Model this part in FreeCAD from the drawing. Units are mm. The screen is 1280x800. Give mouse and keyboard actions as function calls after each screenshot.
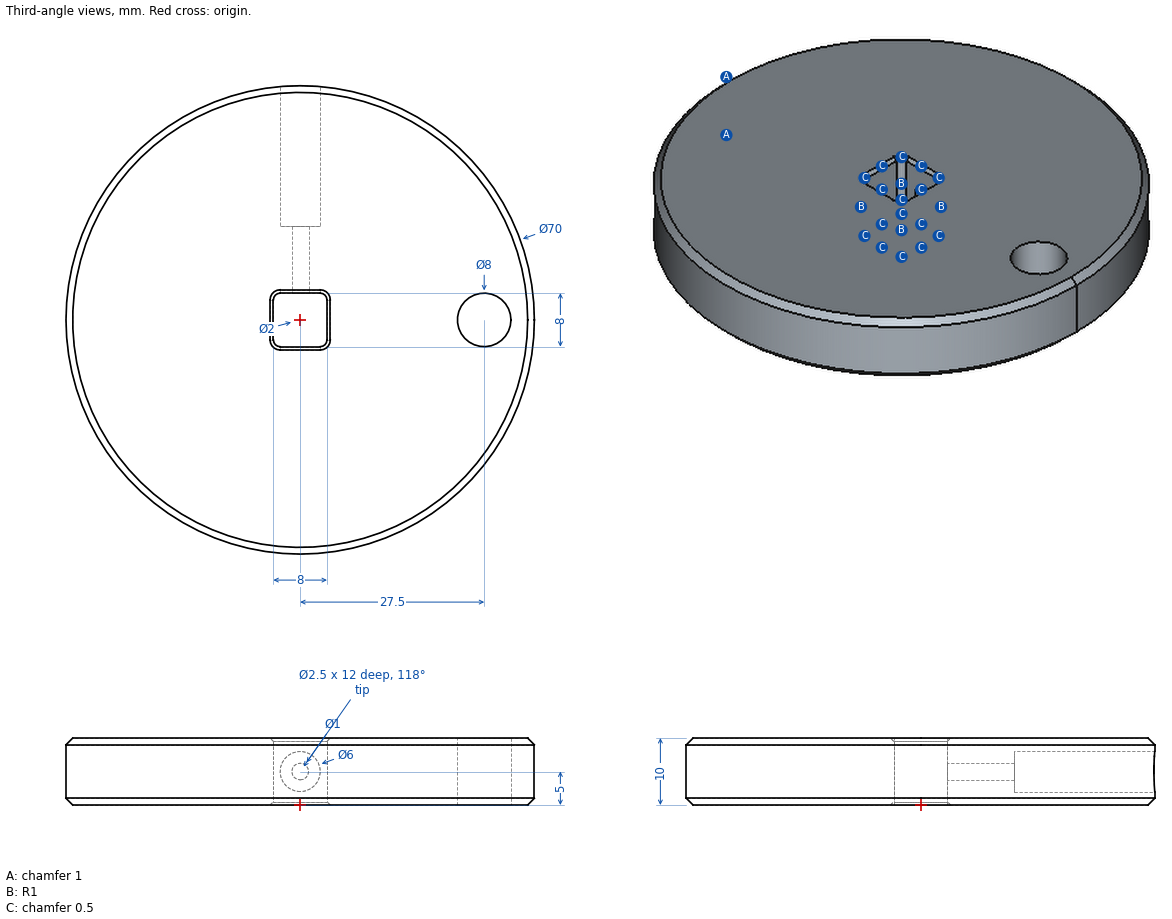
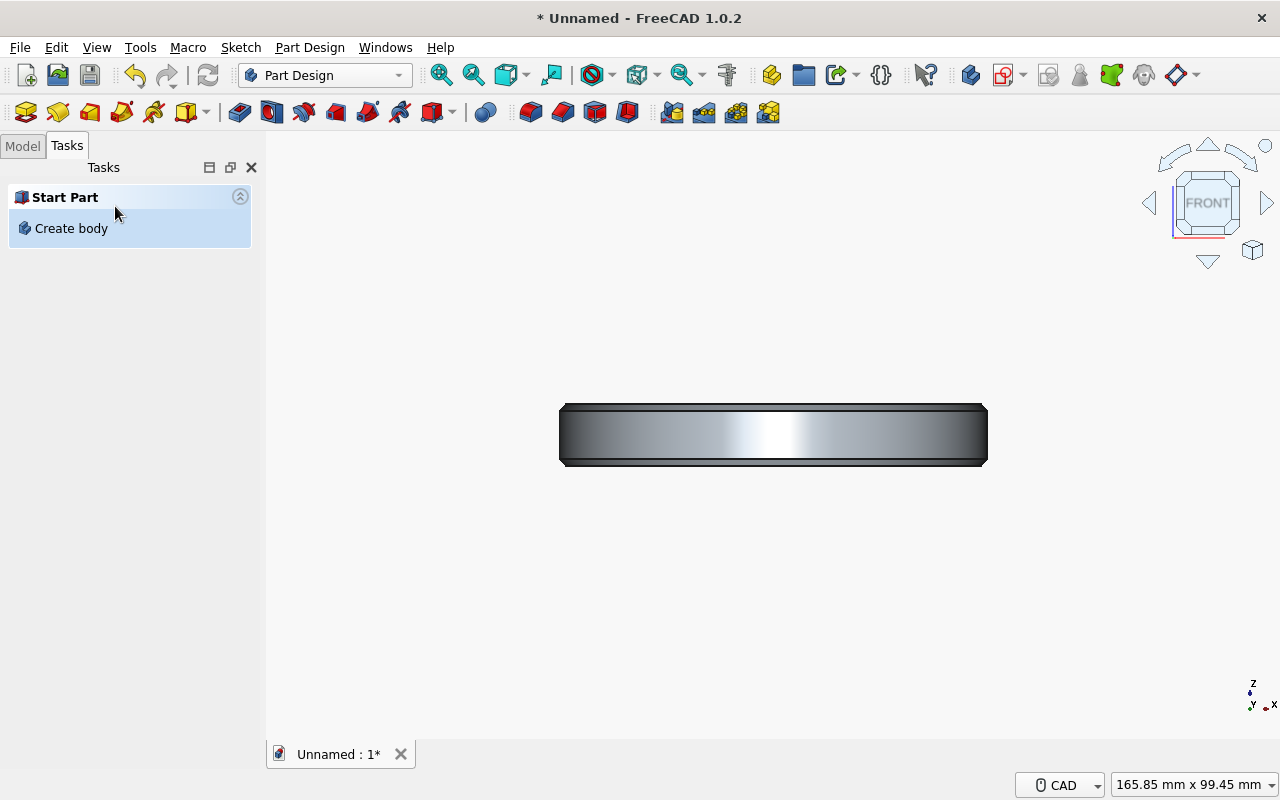
click(442, 76)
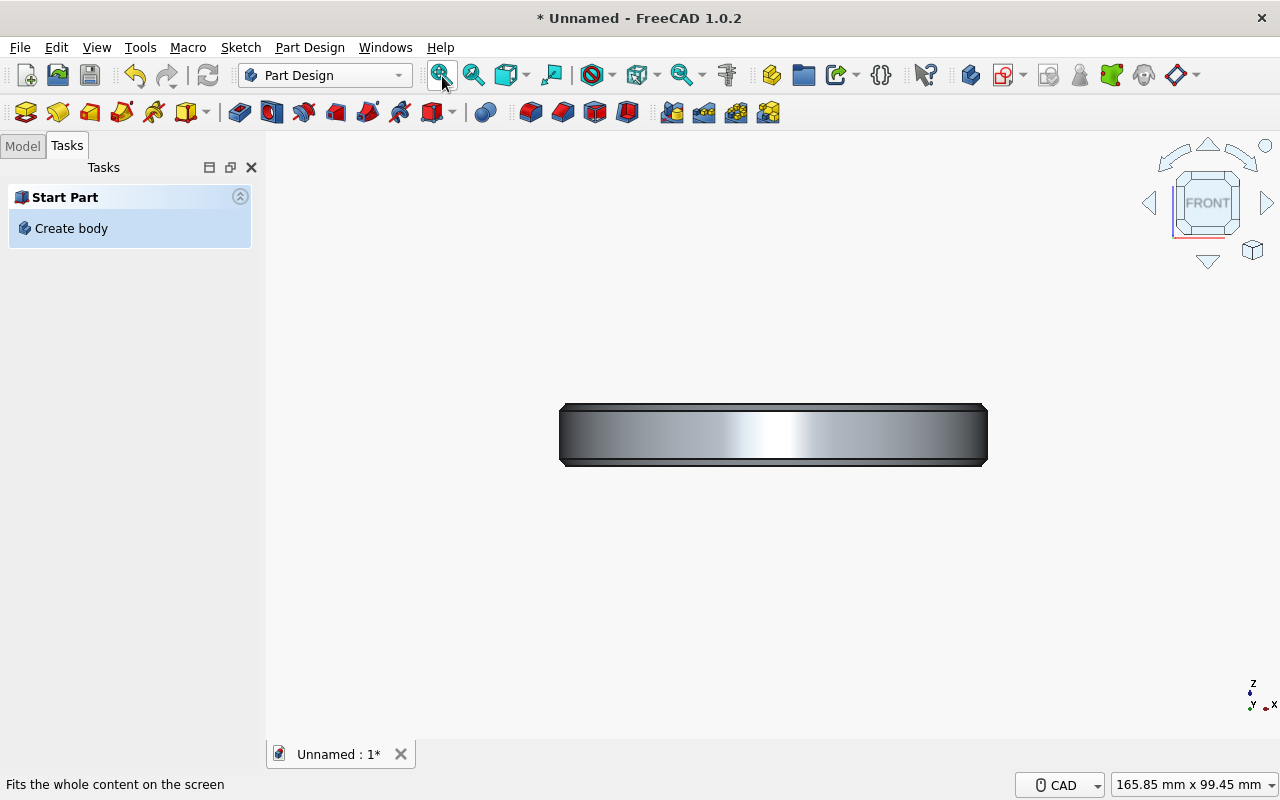
key(3)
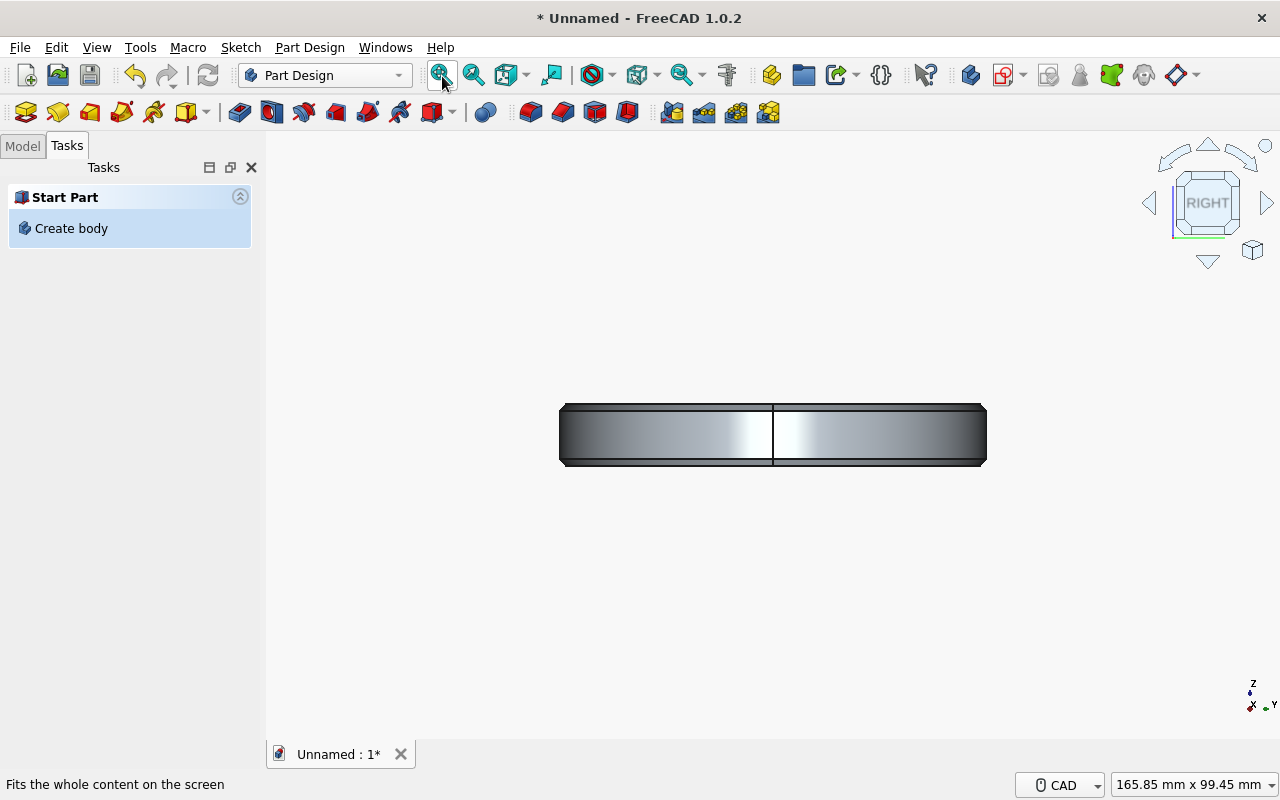
click(442, 76)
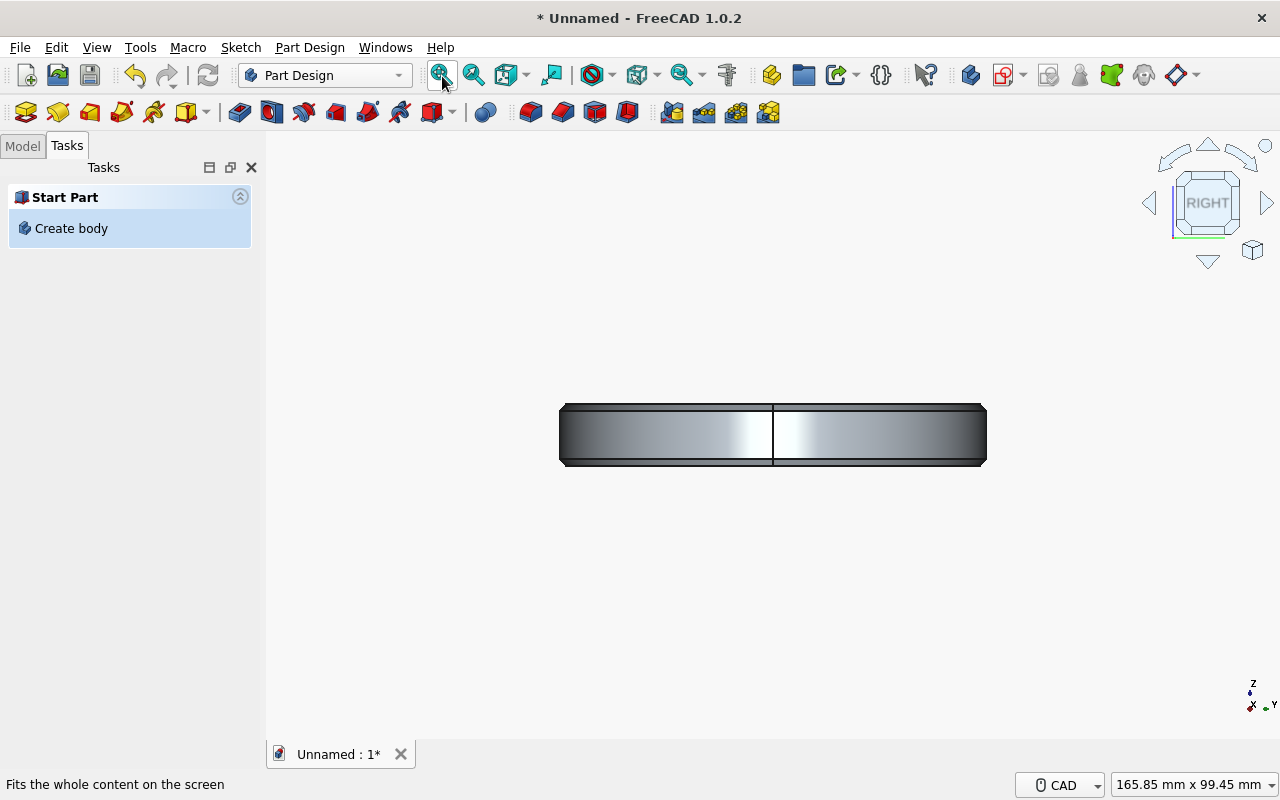
key(5)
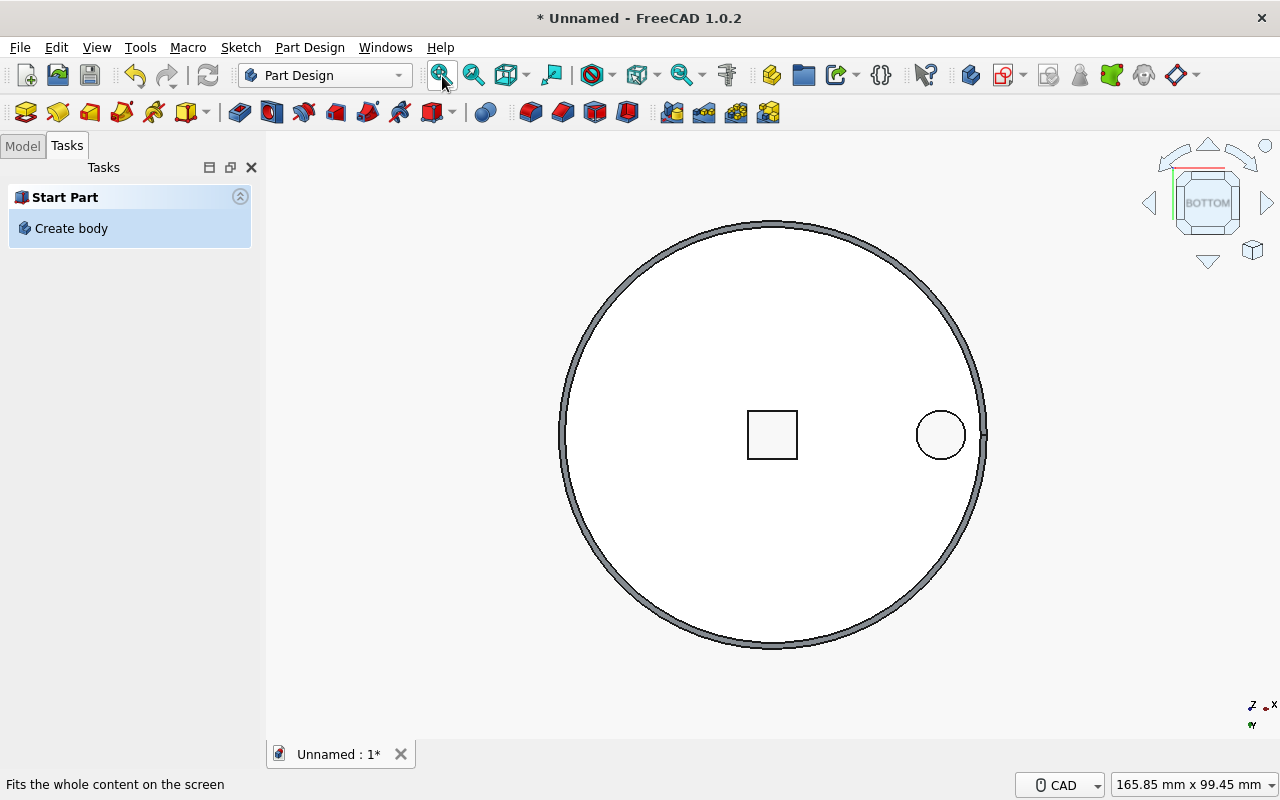
key(4)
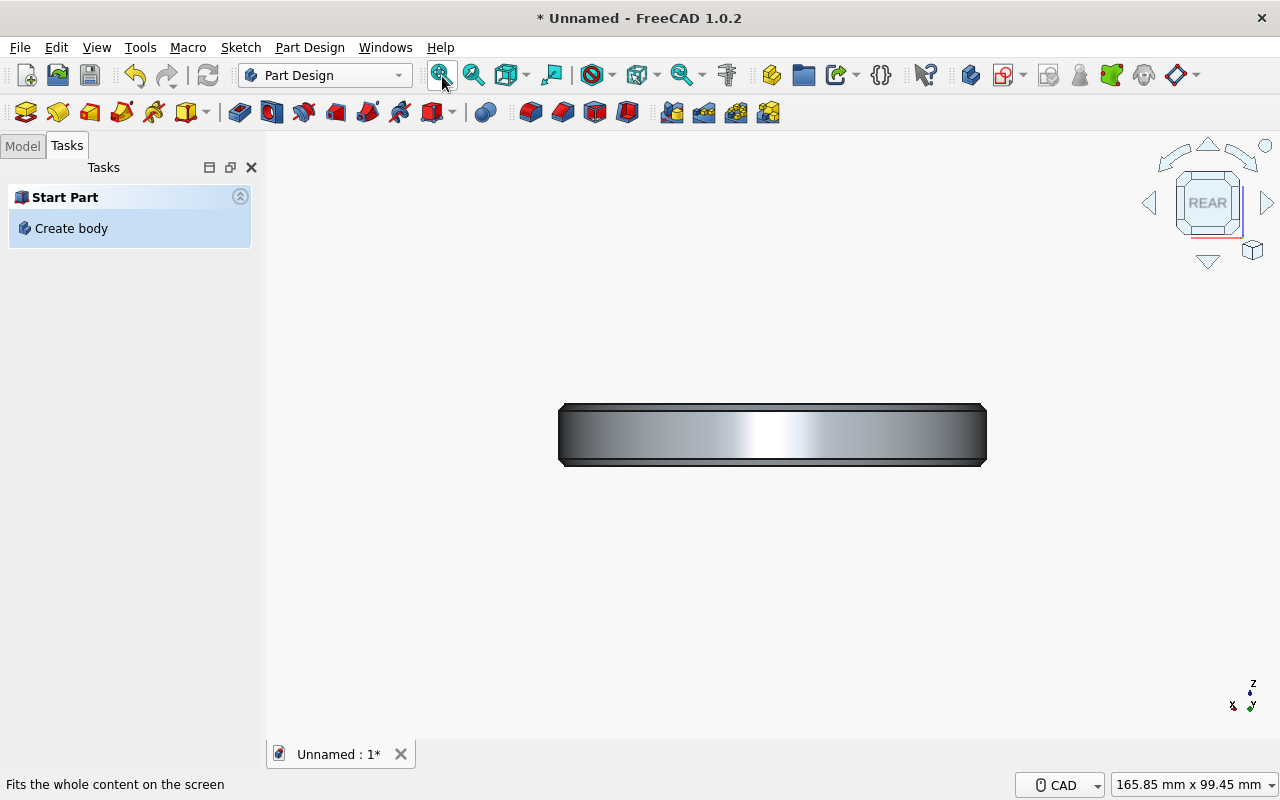
click(442, 76)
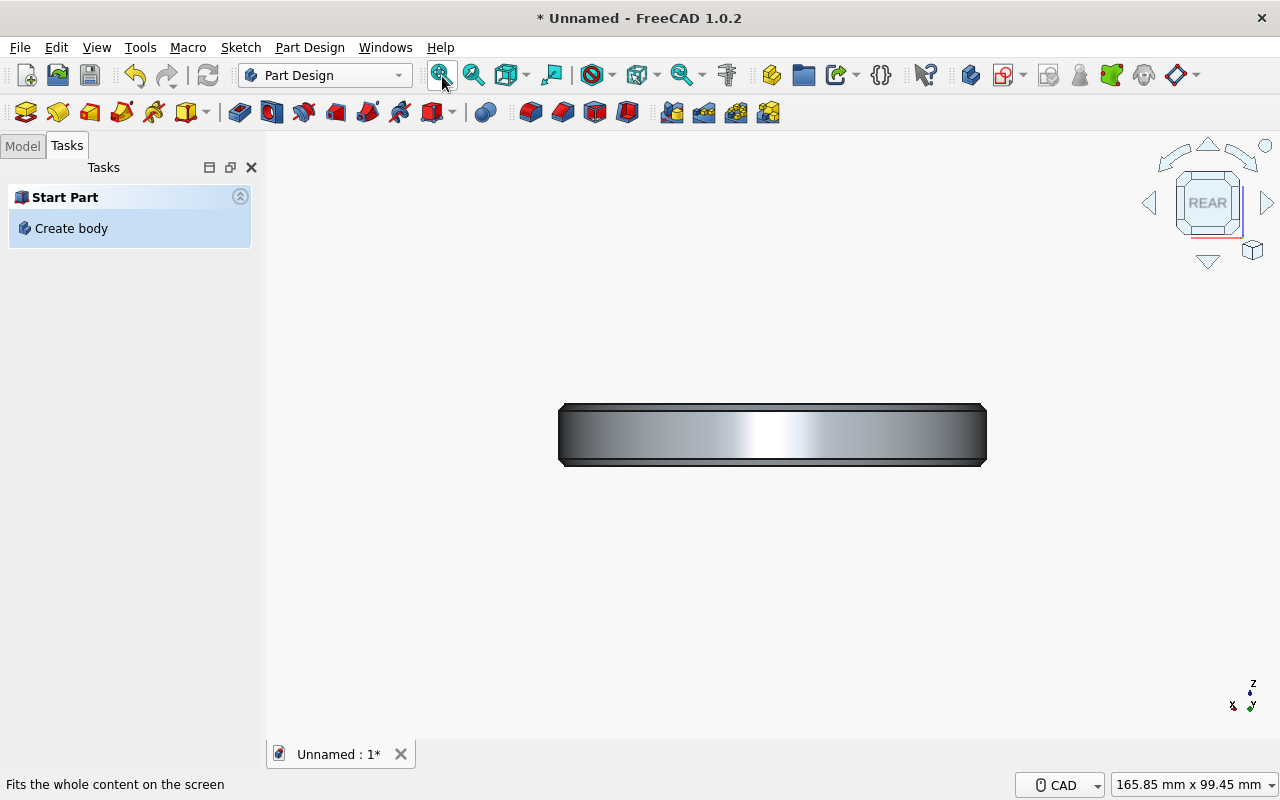
key(6)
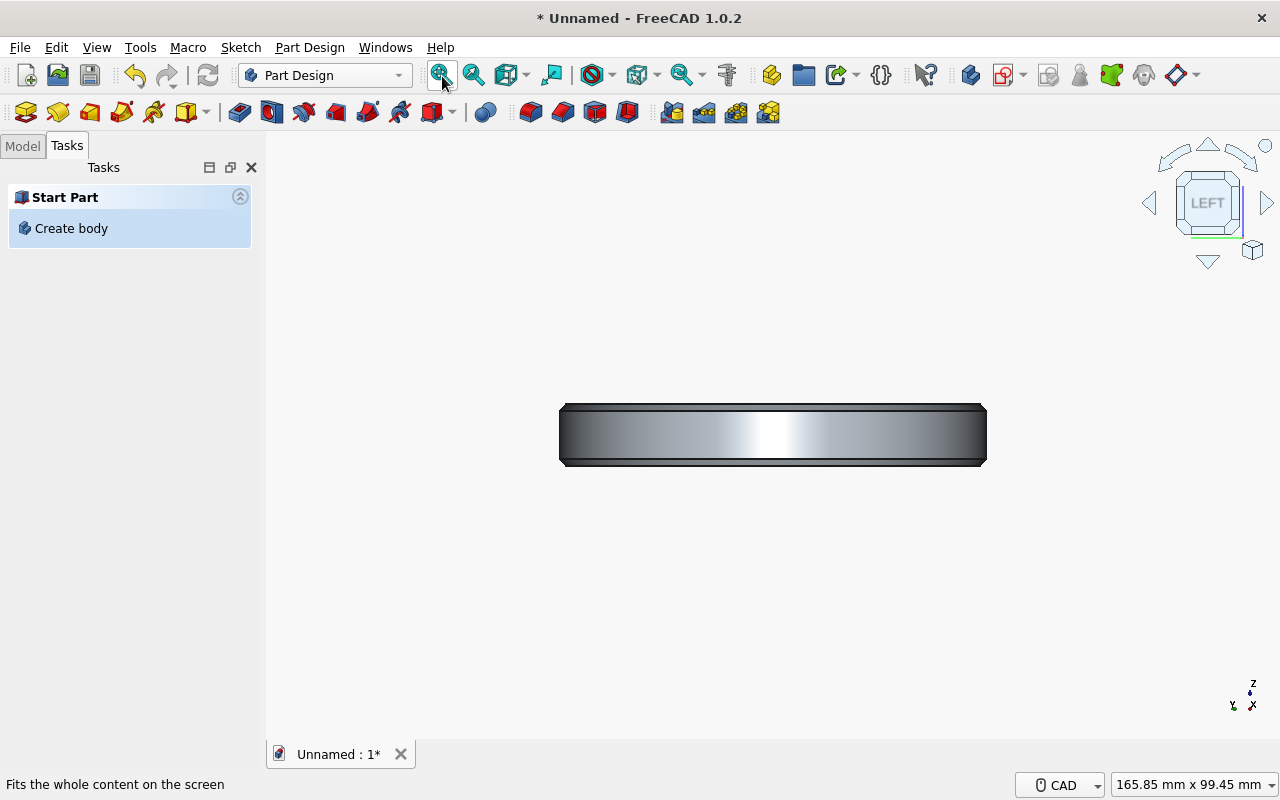
click(442, 76)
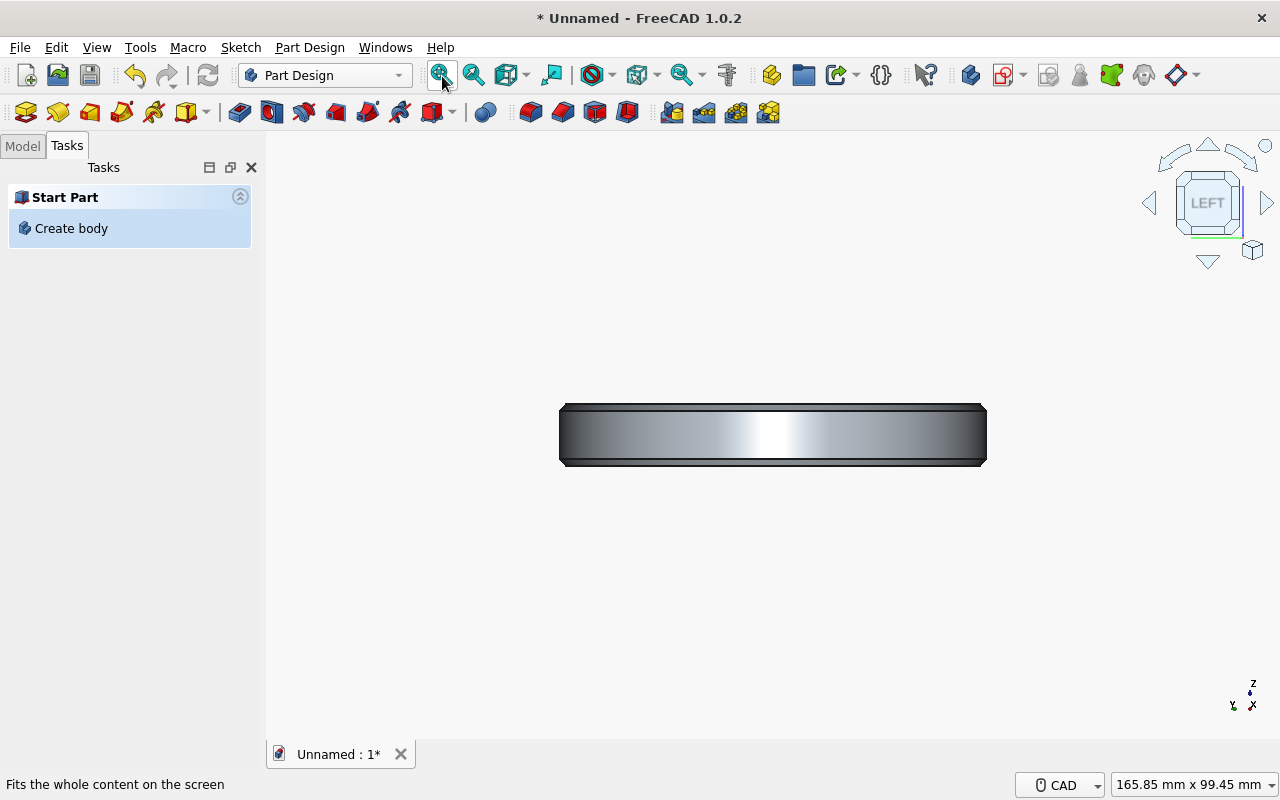
key(v)
key(3)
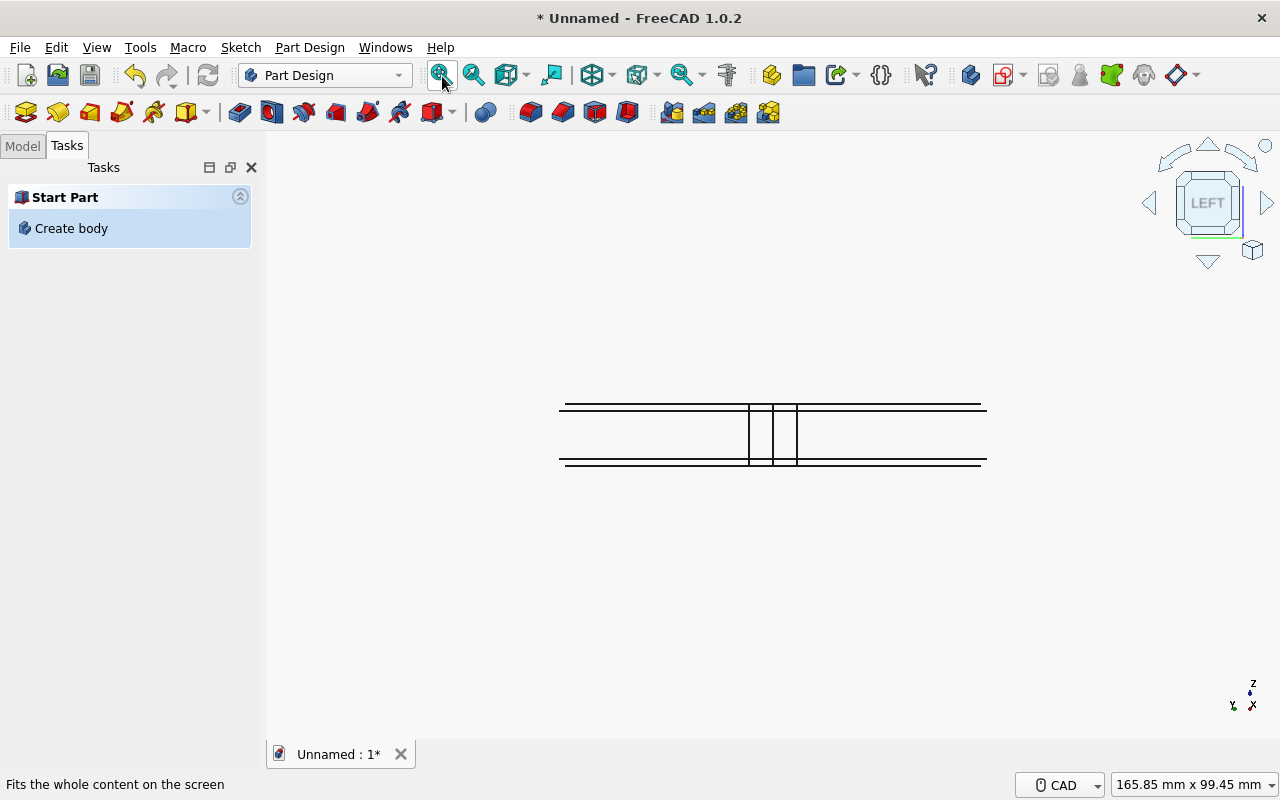
key(0)